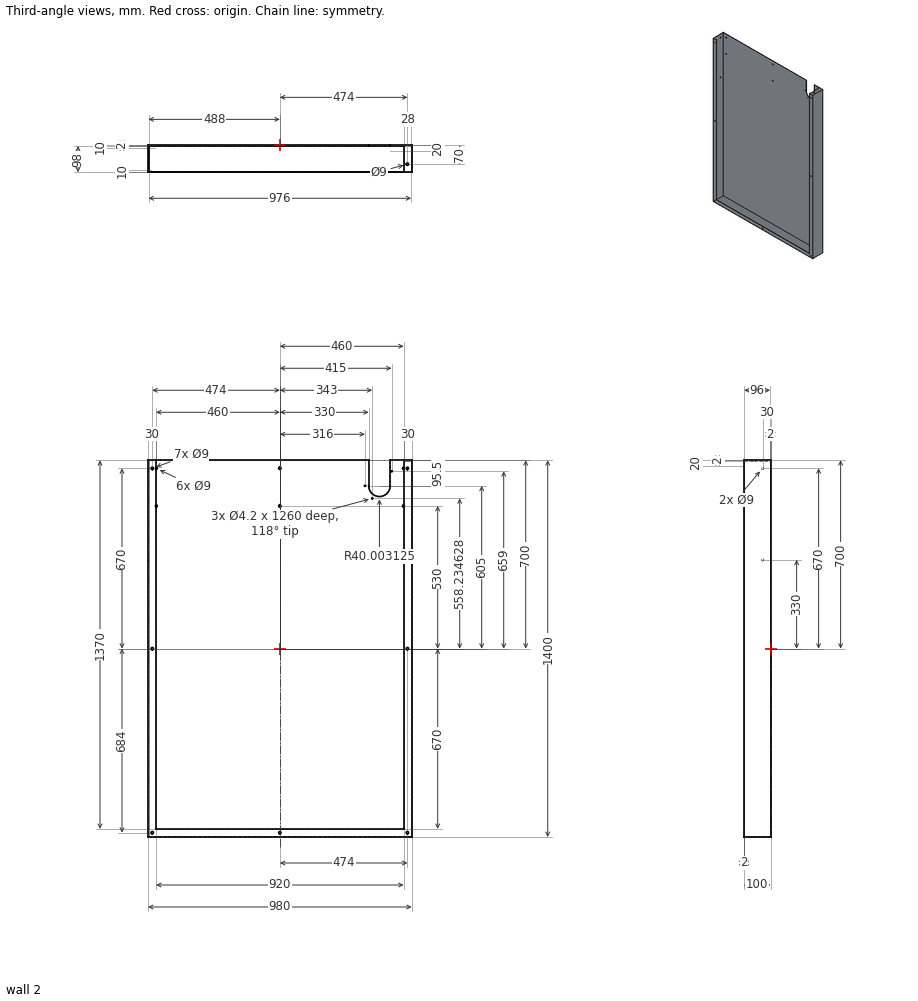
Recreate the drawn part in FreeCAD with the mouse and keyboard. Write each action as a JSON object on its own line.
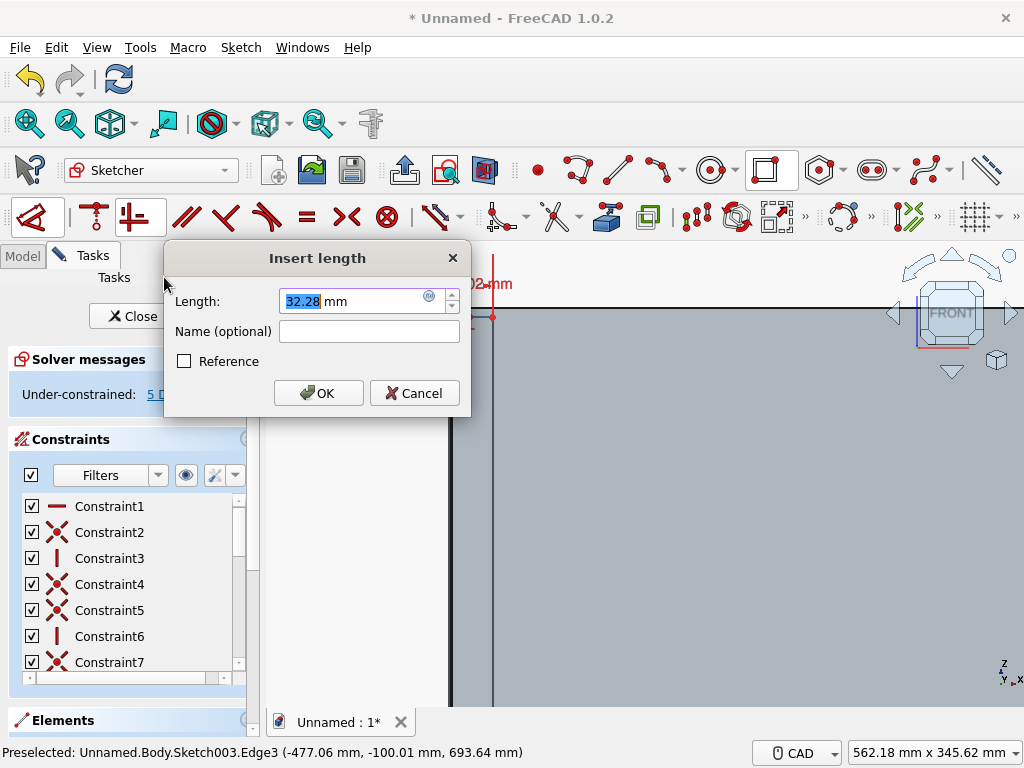
{"action": "type", "text": "30"}
{"action": "key", "text": "Return"}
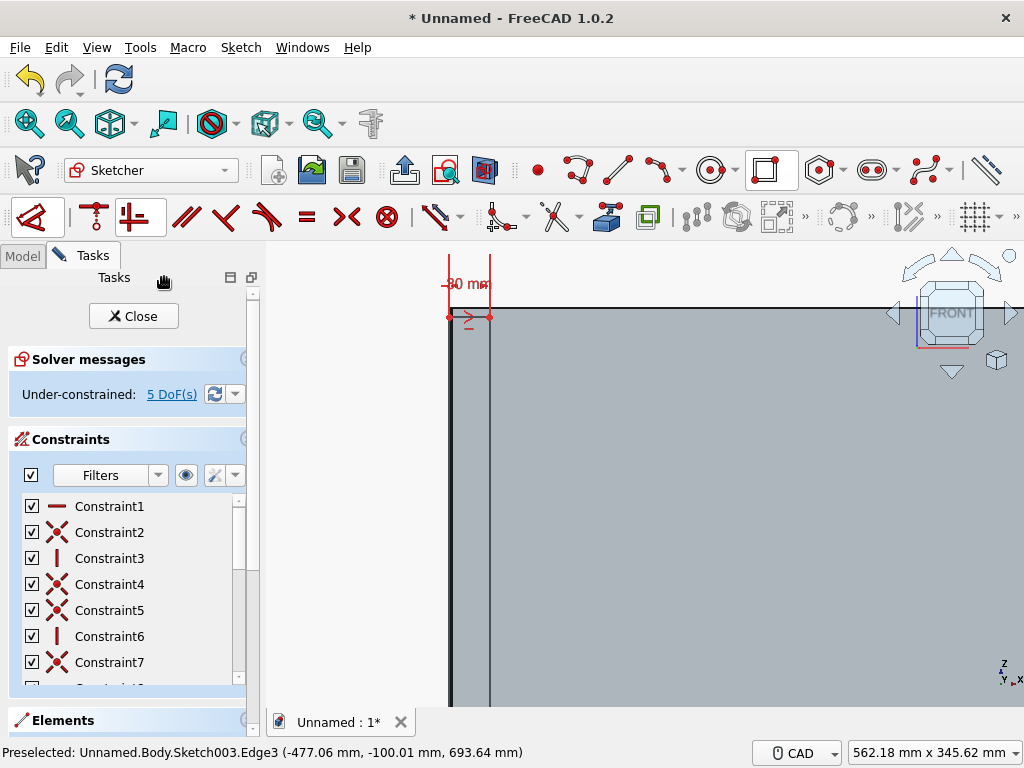
{"action": "scroll", "coordinate": [471, 320], "scroll_direction": "down", "scroll_amount": 9}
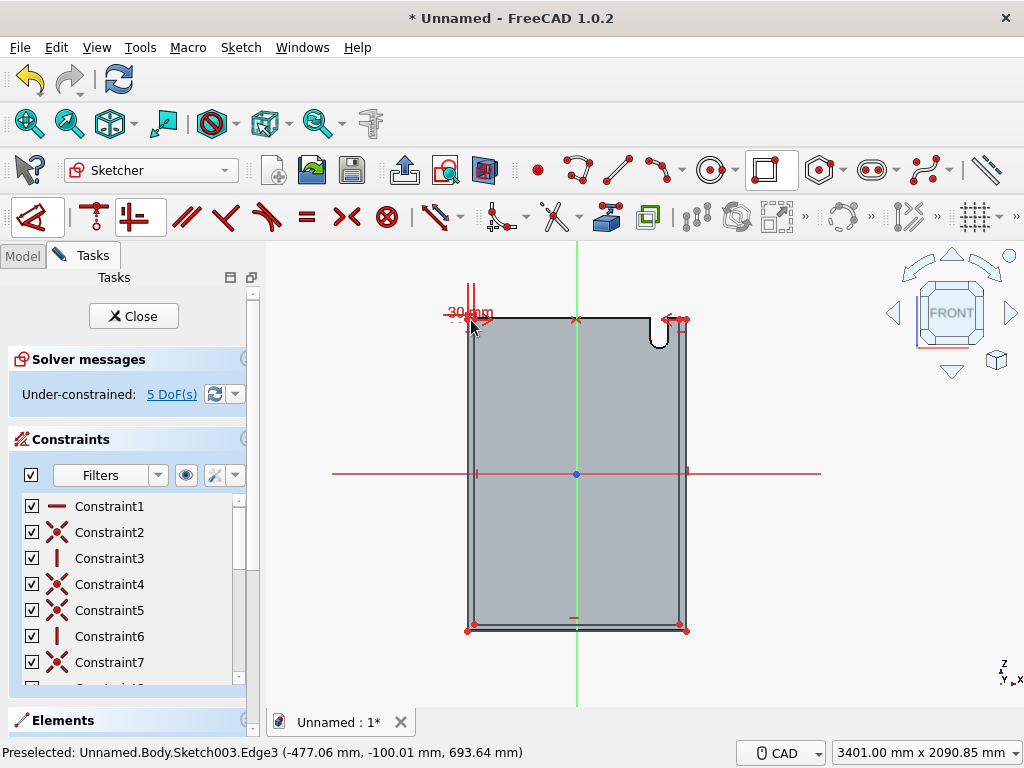
{"action": "scroll", "coordinate": [684, 320], "scroll_direction": "up", "scroll_amount": 10}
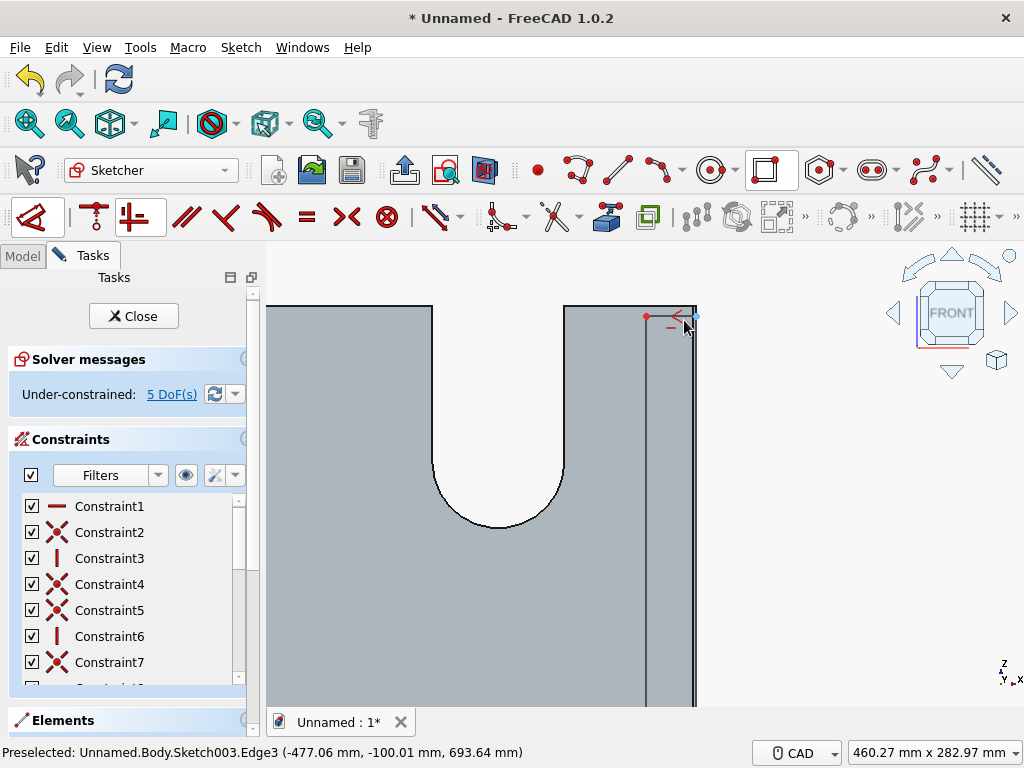
{"action": "left_click", "coordinate": [681, 316]}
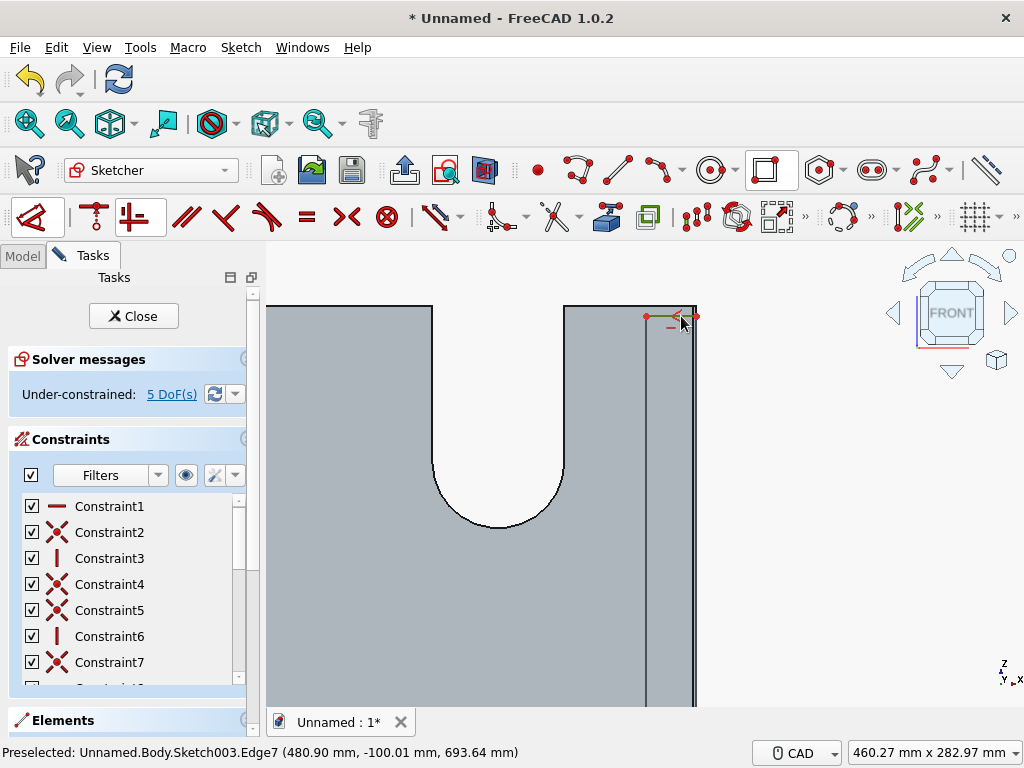
{"action": "key", "text": "l"}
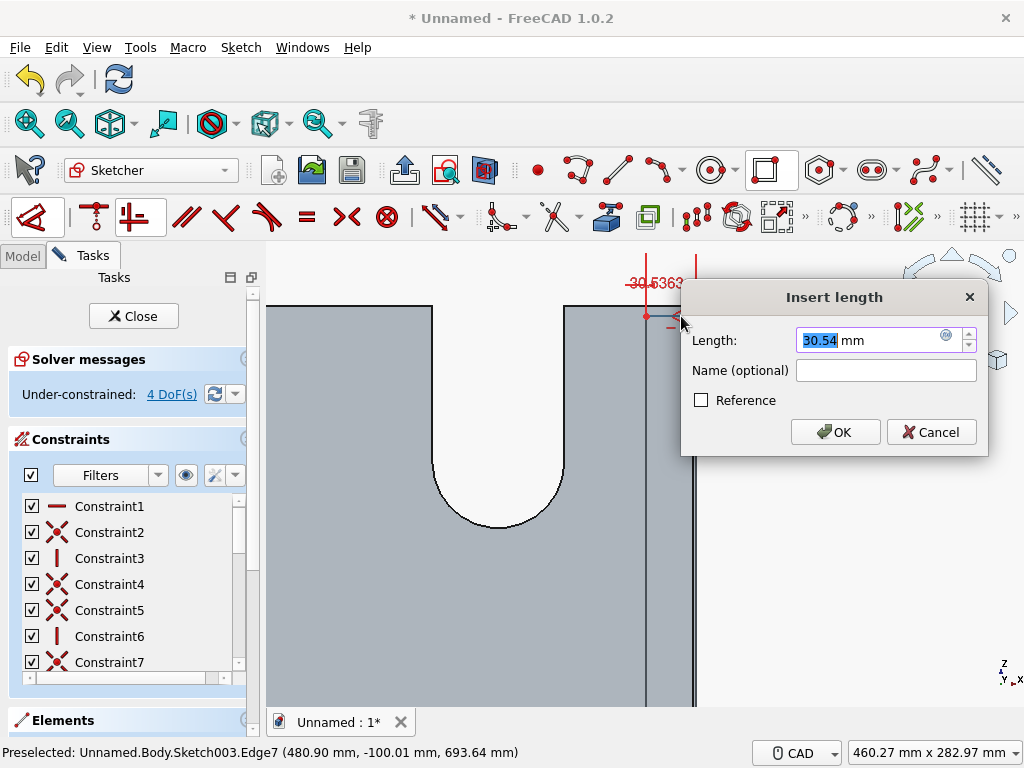
{"action": "type", "text": "30"}
{"action": "key", "text": "Return"}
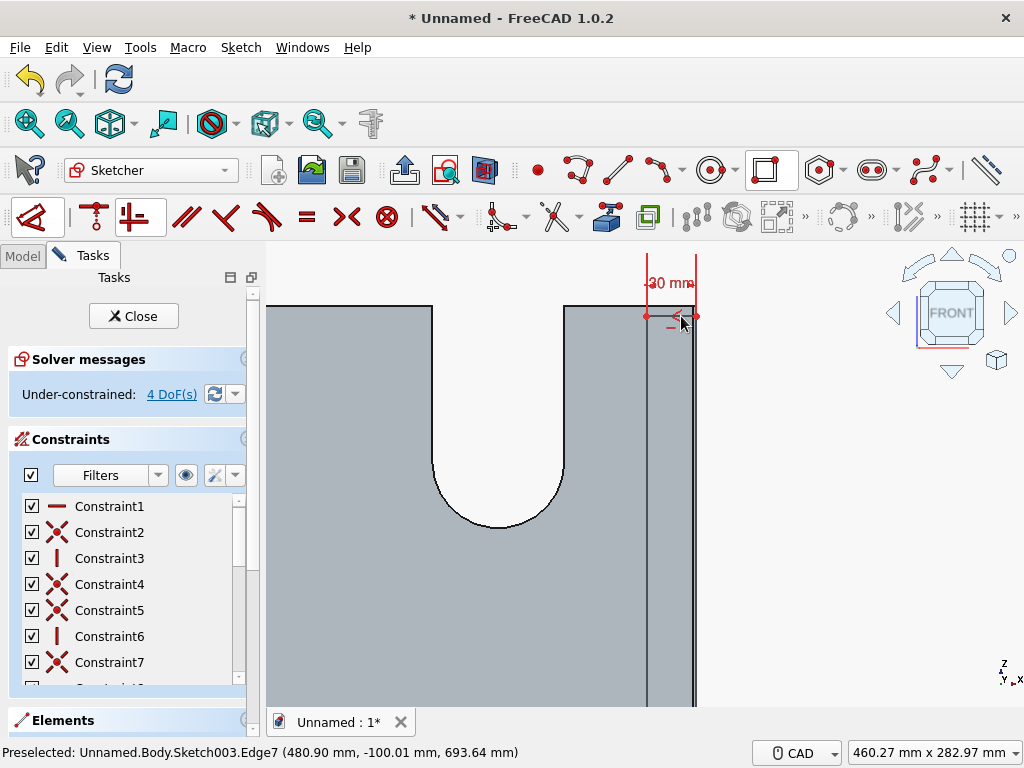
{"action": "scroll", "coordinate": [684, 320], "scroll_direction": "down", "scroll_amount": 10}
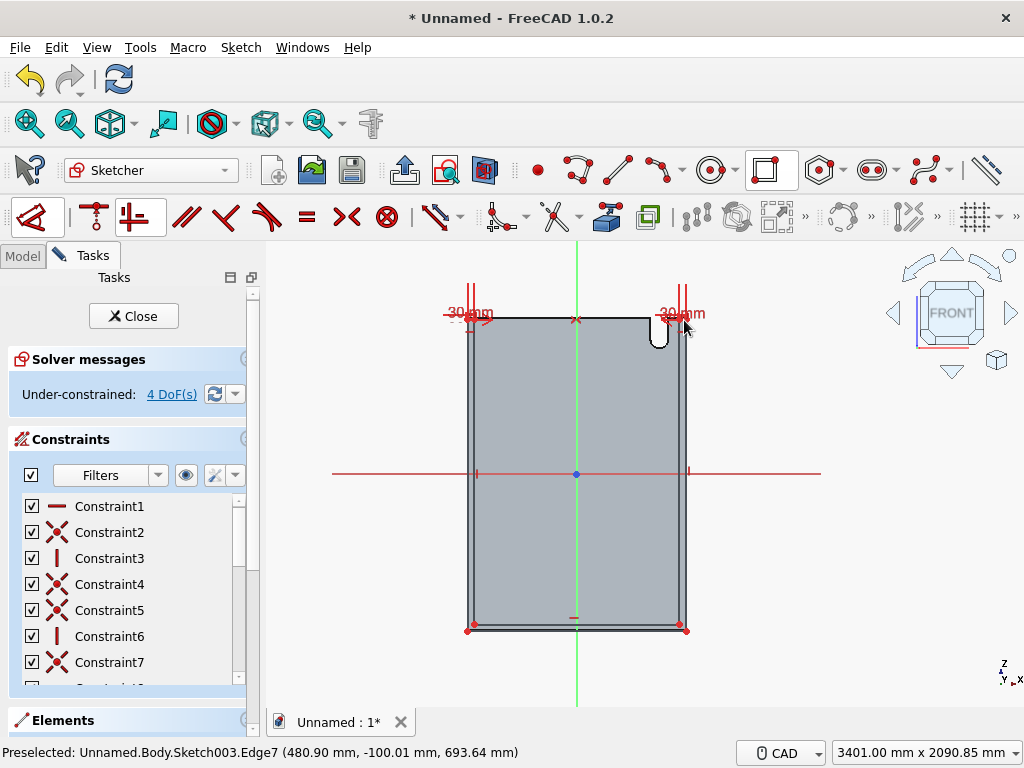
{"action": "scroll", "coordinate": [618, 625], "scroll_direction": "up", "scroll_amount": 4}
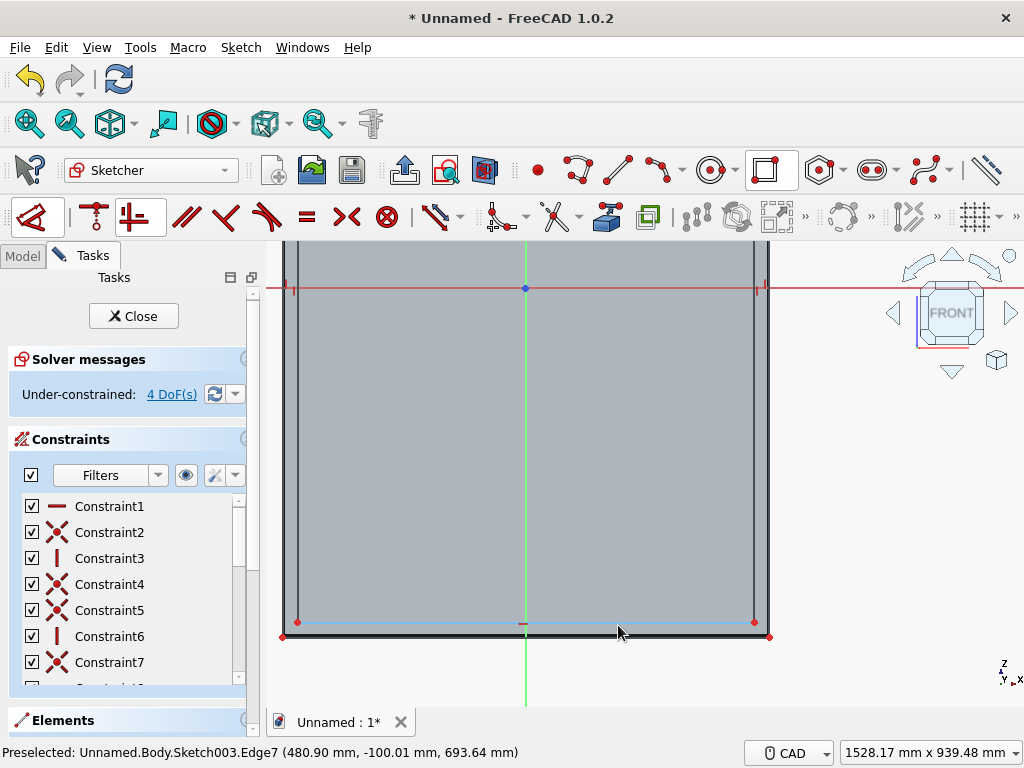
{"action": "left_click", "coordinate": [617, 623]}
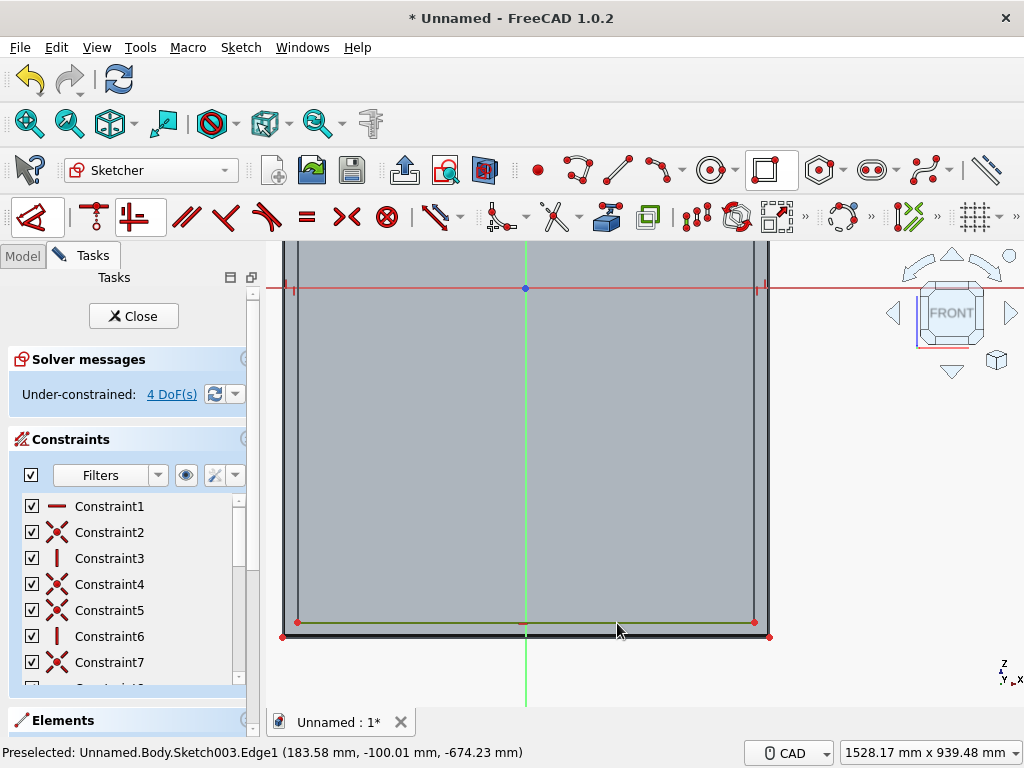
{"action": "key", "text": "l"}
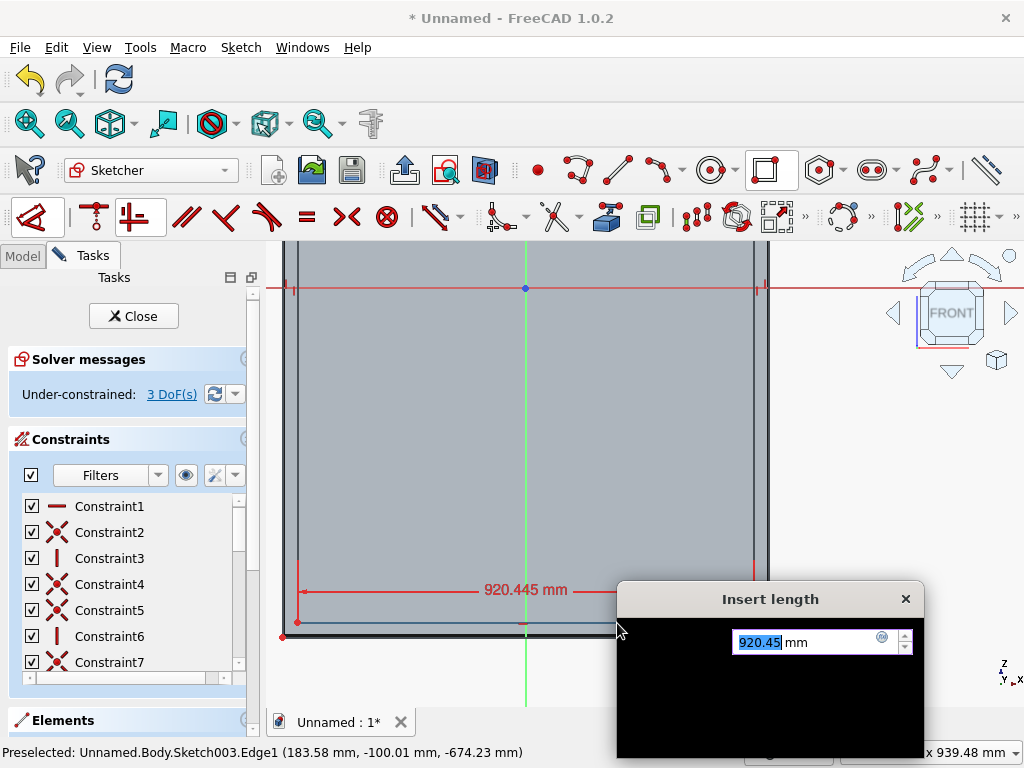
{"action": "type", "text": "920"}
{"action": "key", "text": "Return"}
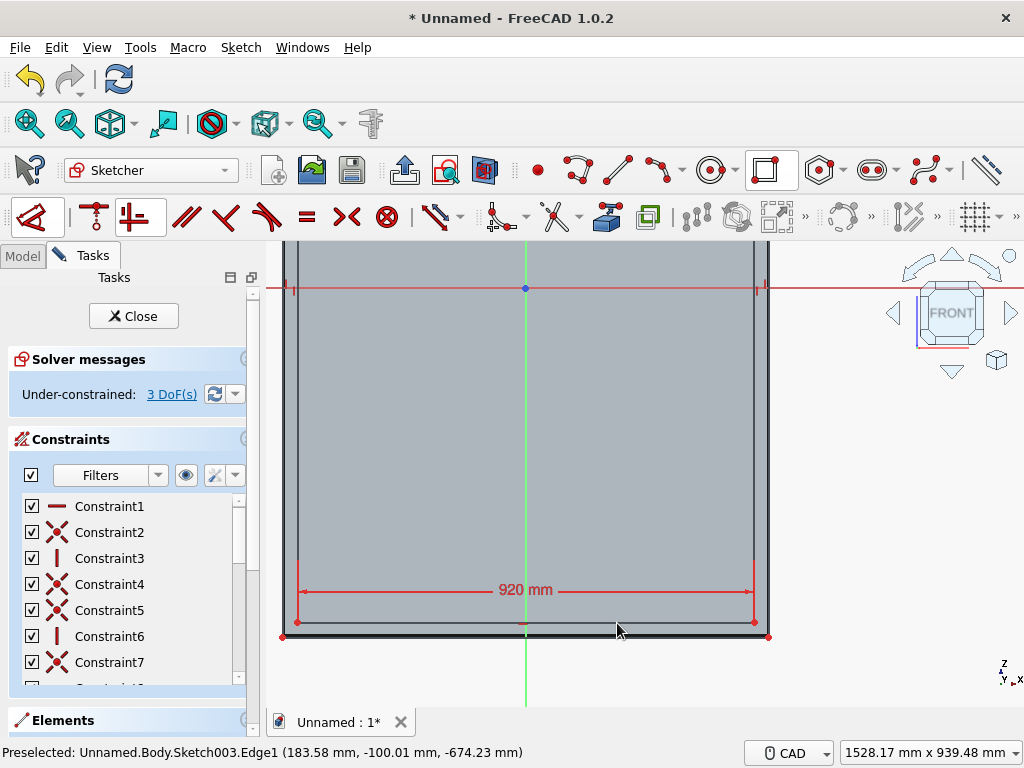
{"action": "left_click", "coordinate": [298, 419]}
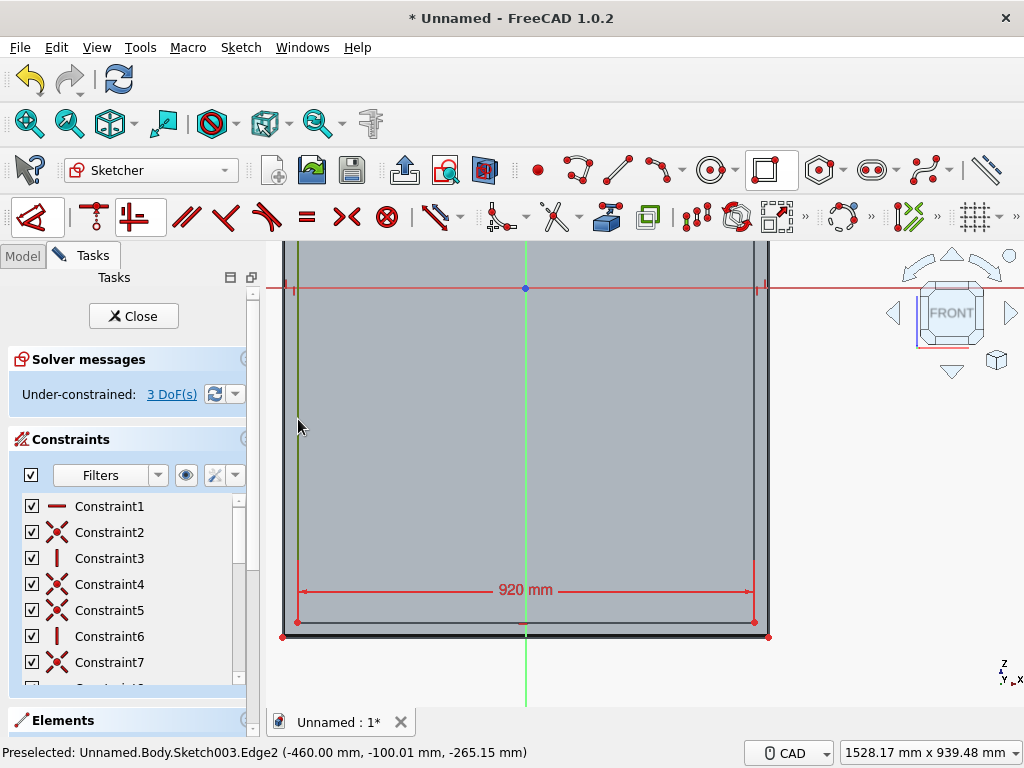
{"action": "key", "text": "i"}